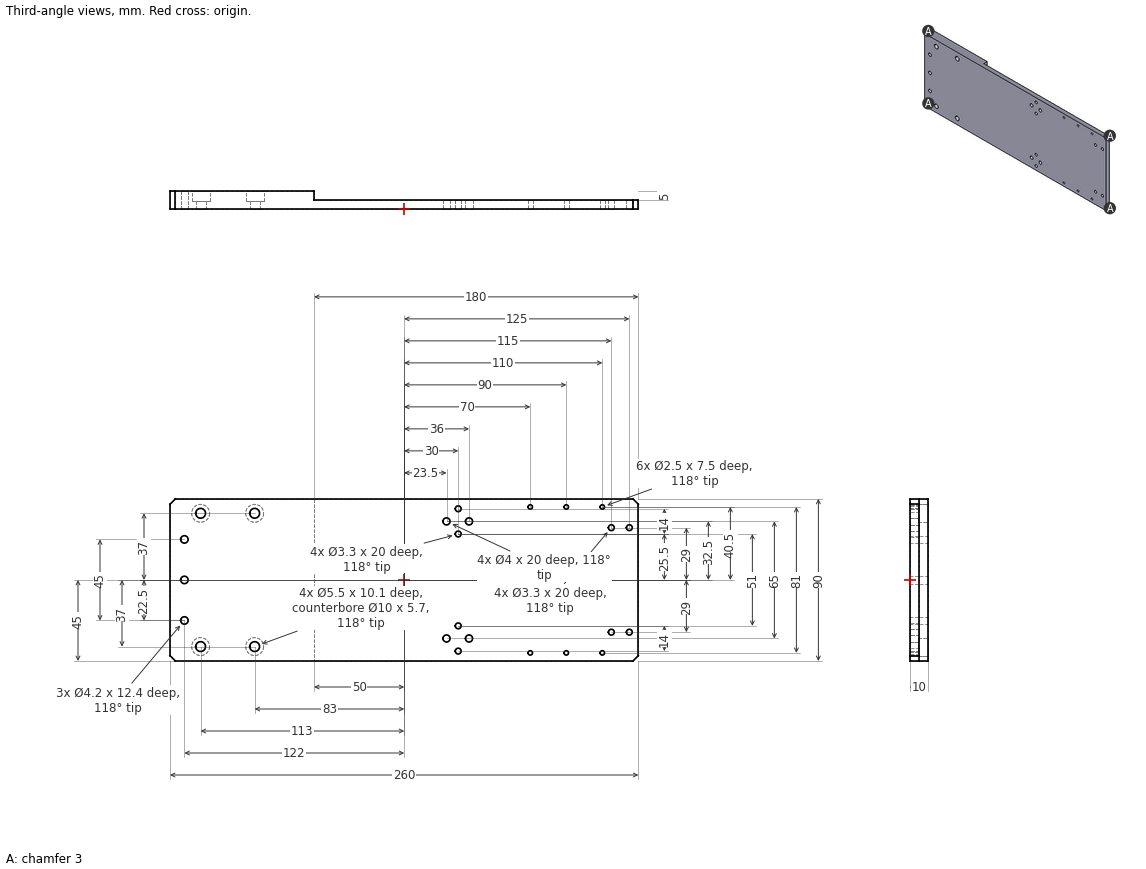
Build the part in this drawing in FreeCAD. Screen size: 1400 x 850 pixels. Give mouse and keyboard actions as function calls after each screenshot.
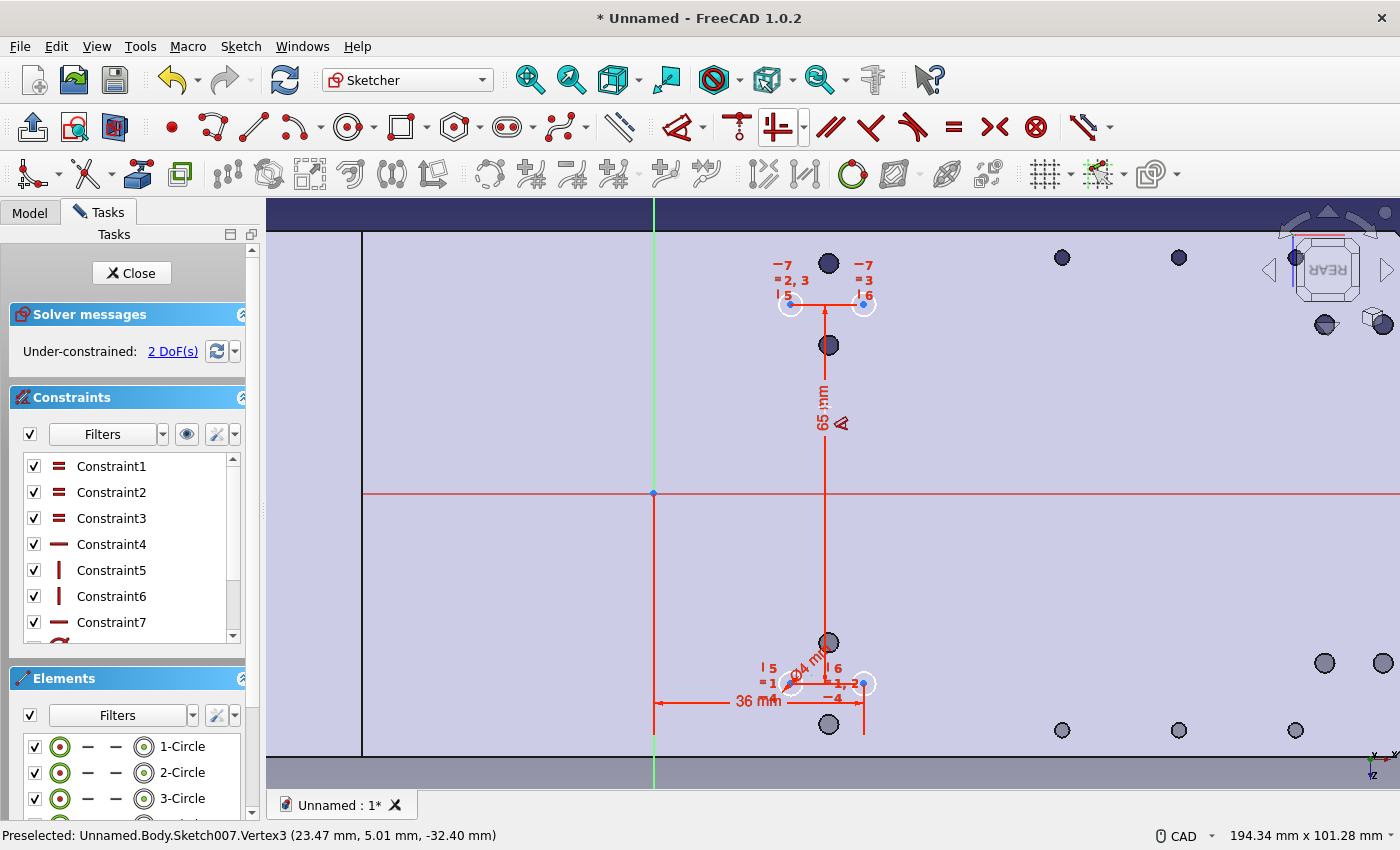
click(791, 684)
click(674, 718)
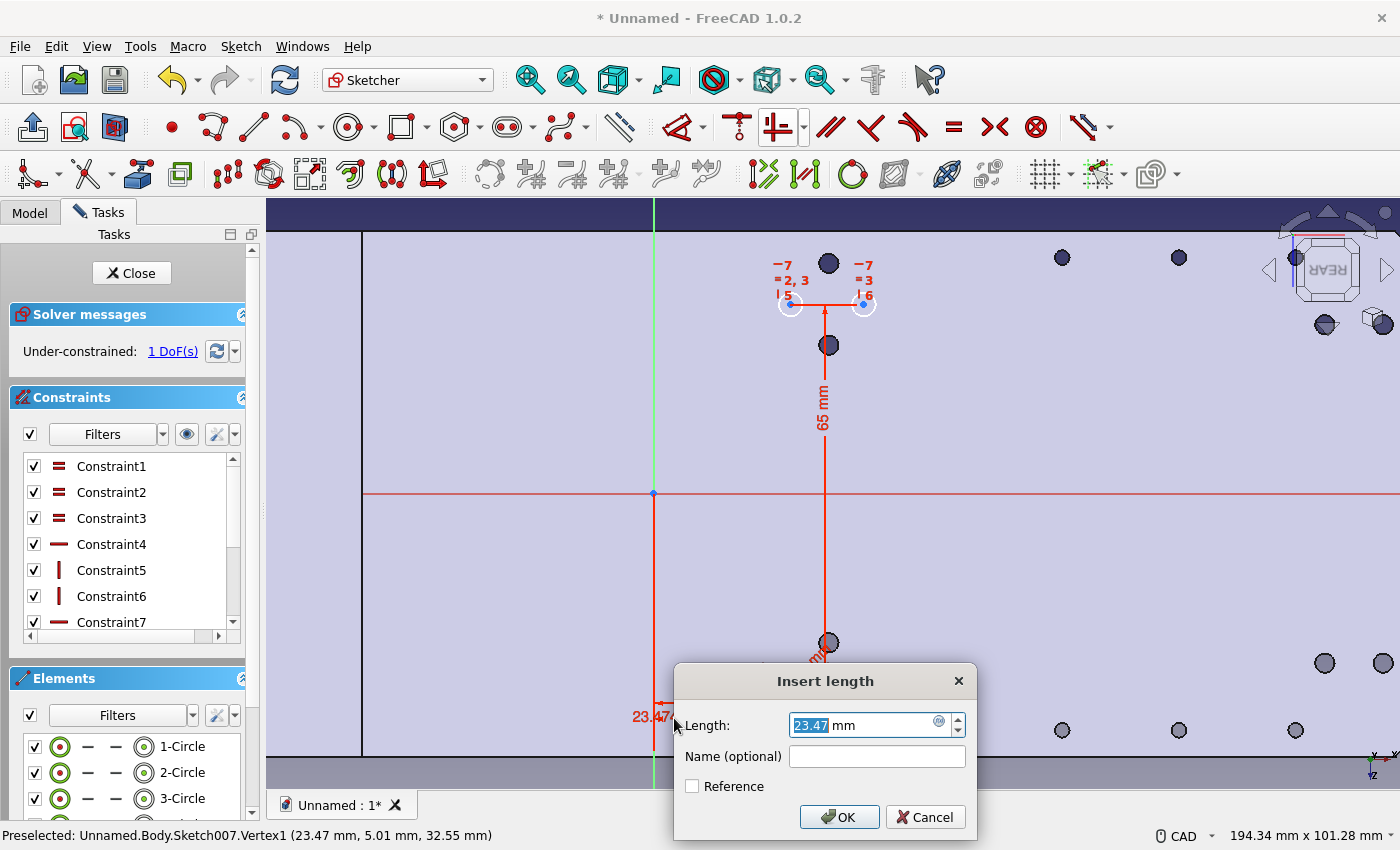
text(23.5)
key(Return)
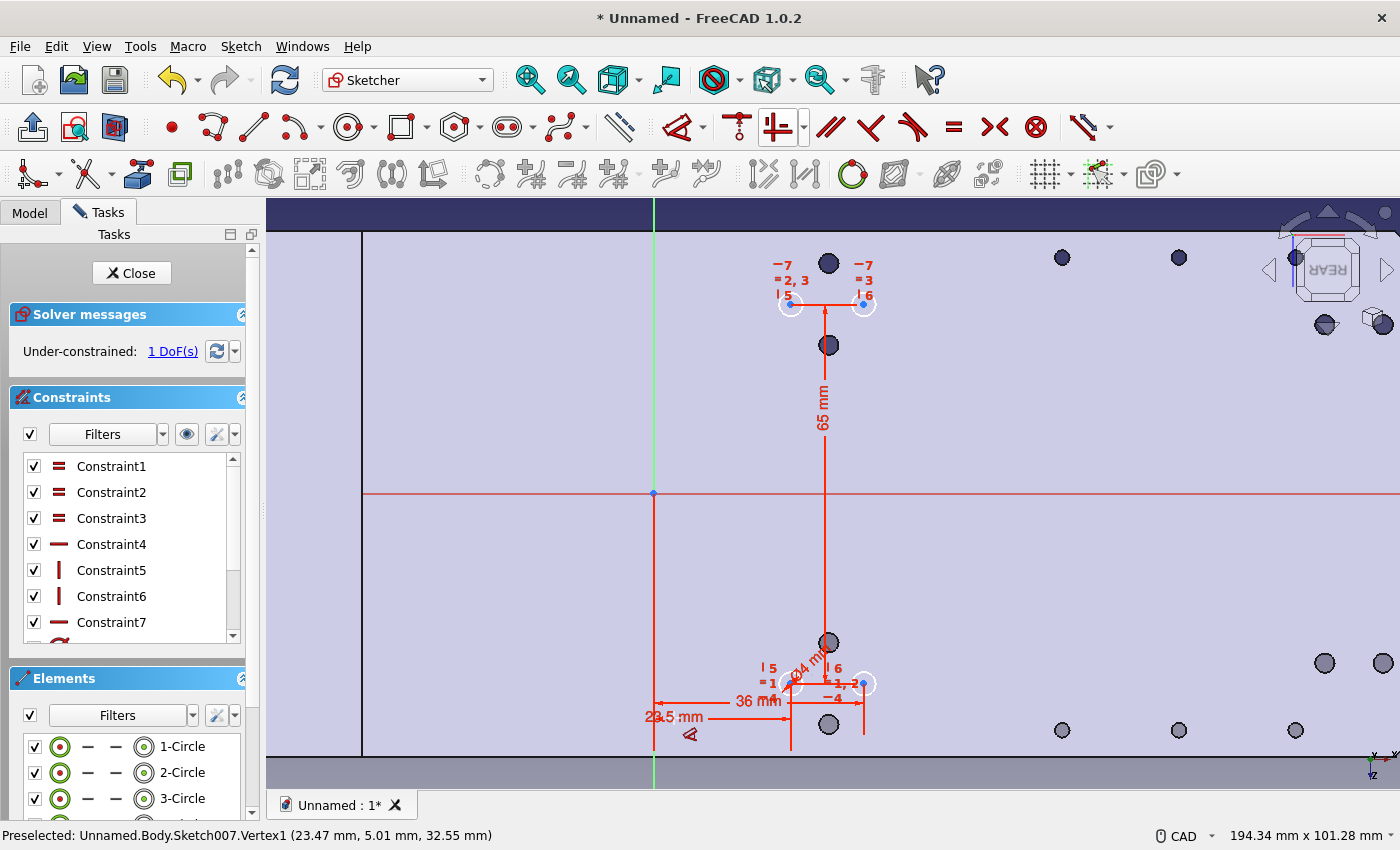
click(791, 684)
click(620, 589)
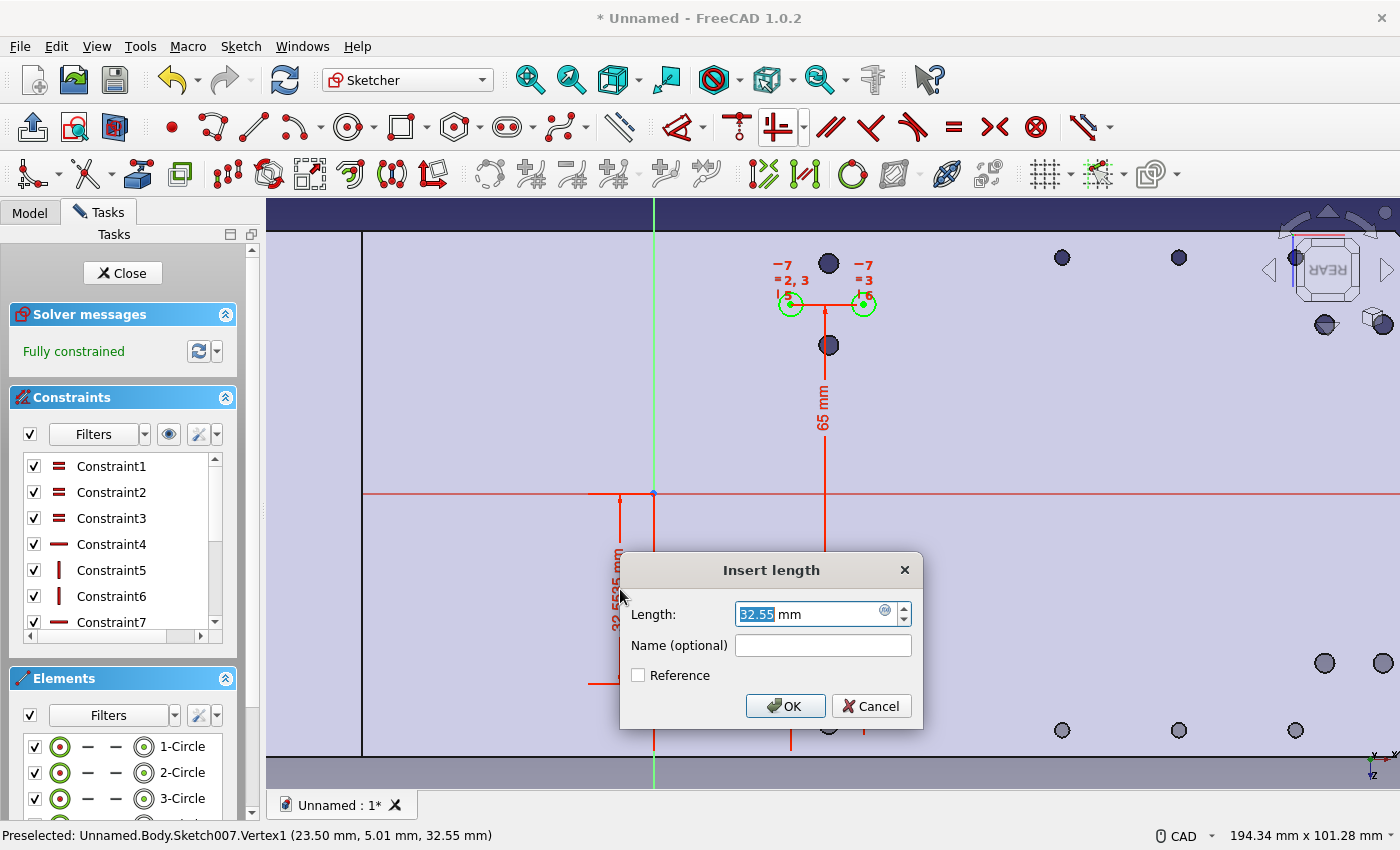
text(32.5)
key(Return)
key(Escape)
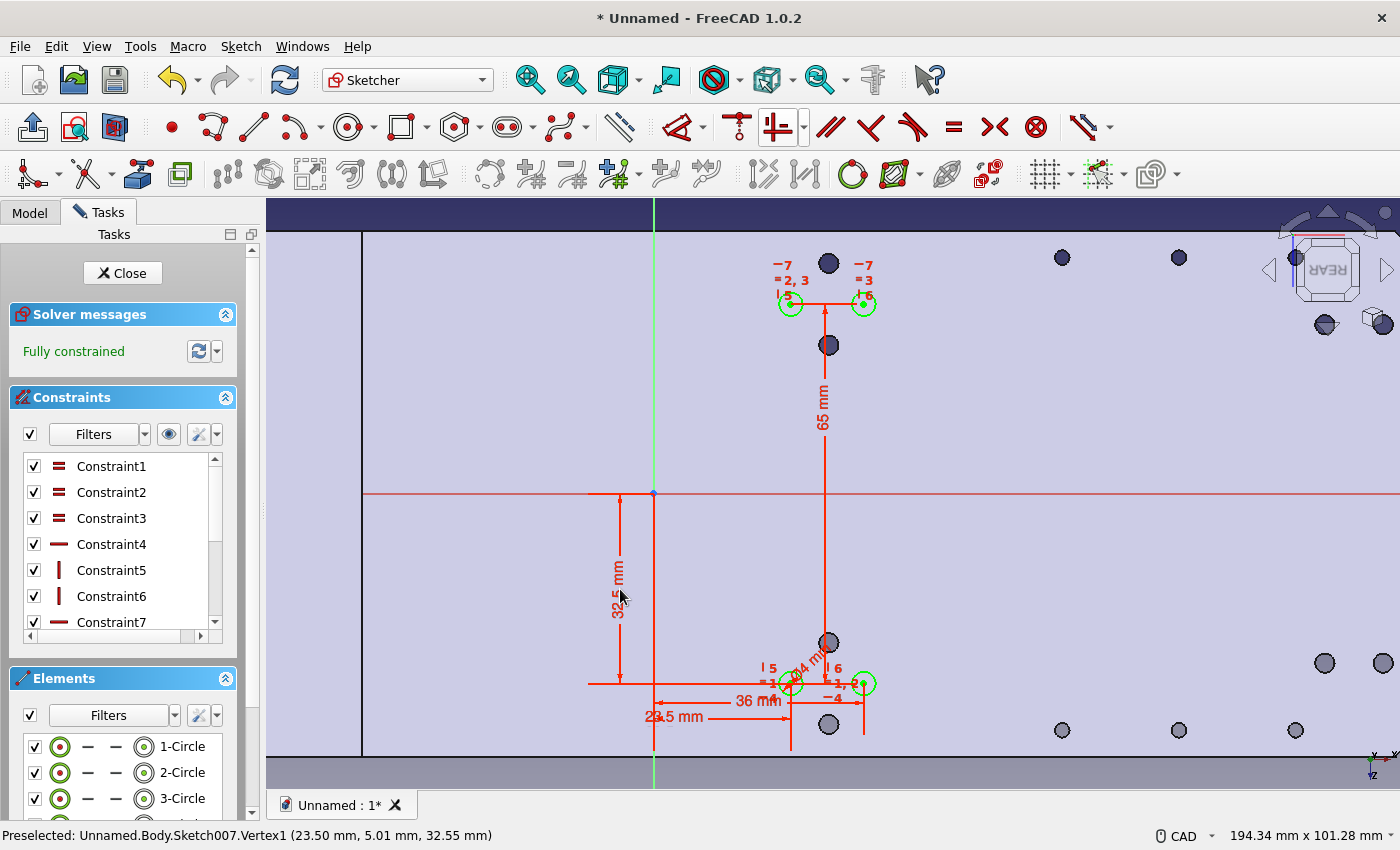
click(123, 273)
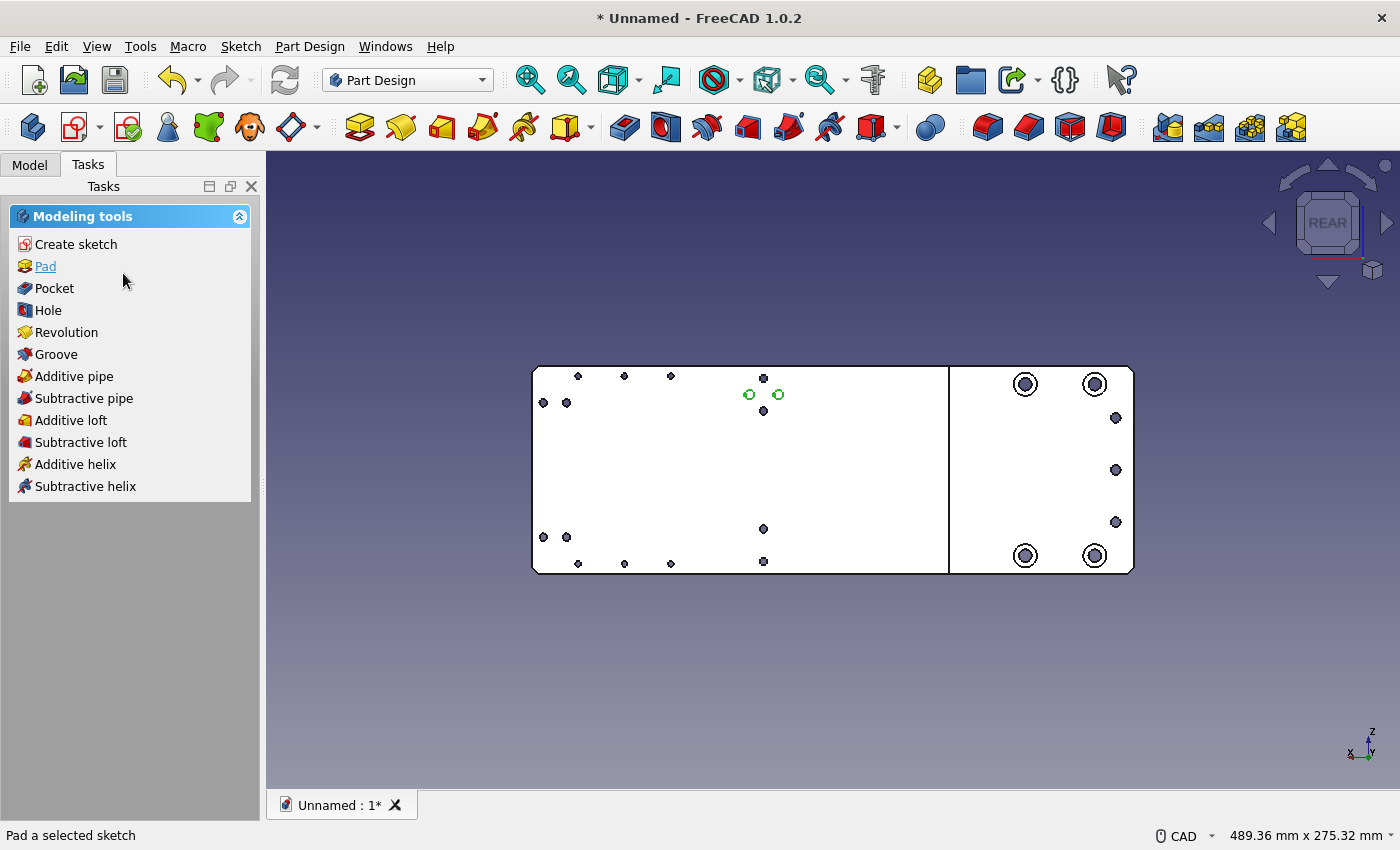
click(666, 128)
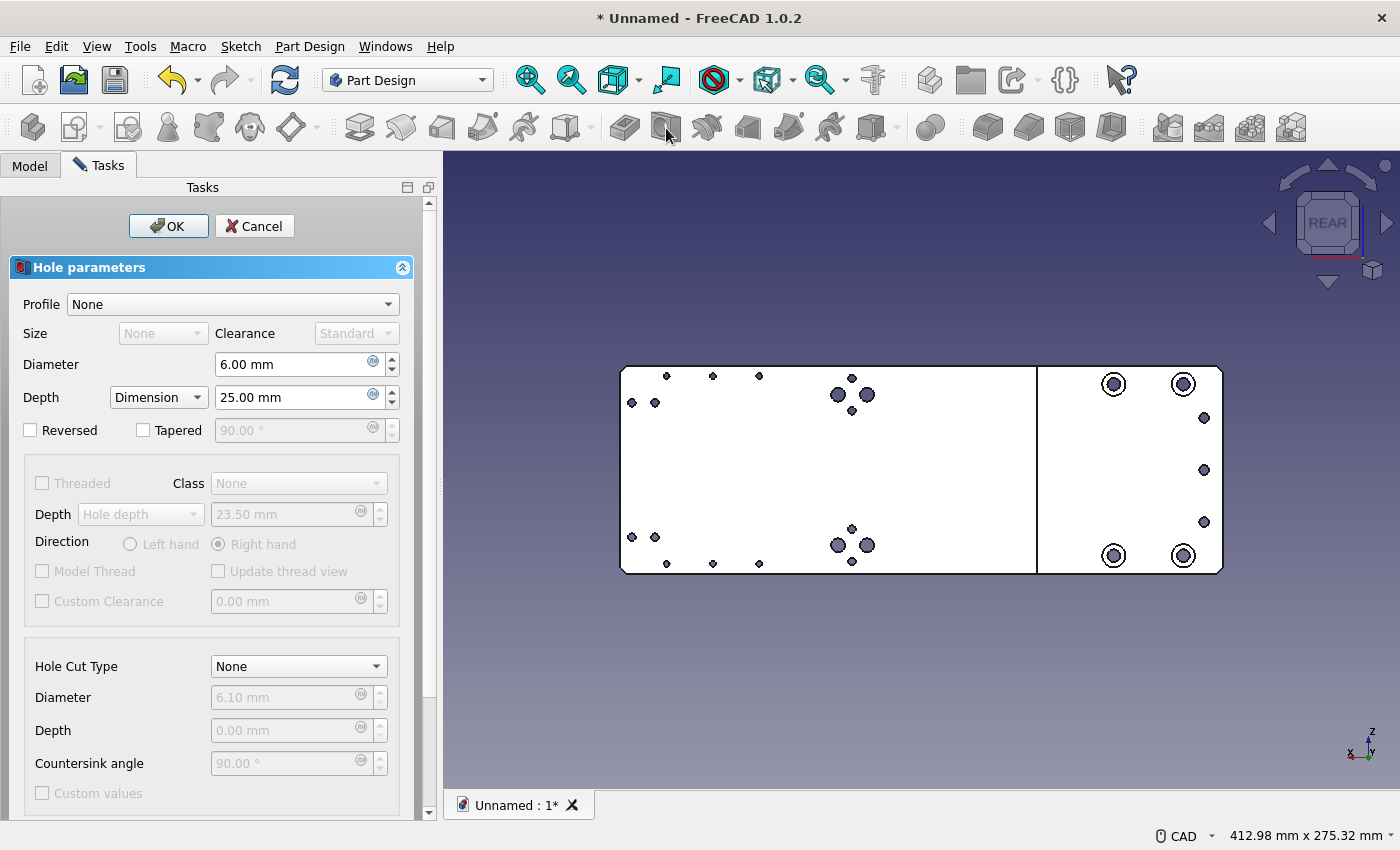
triple_click(300, 364)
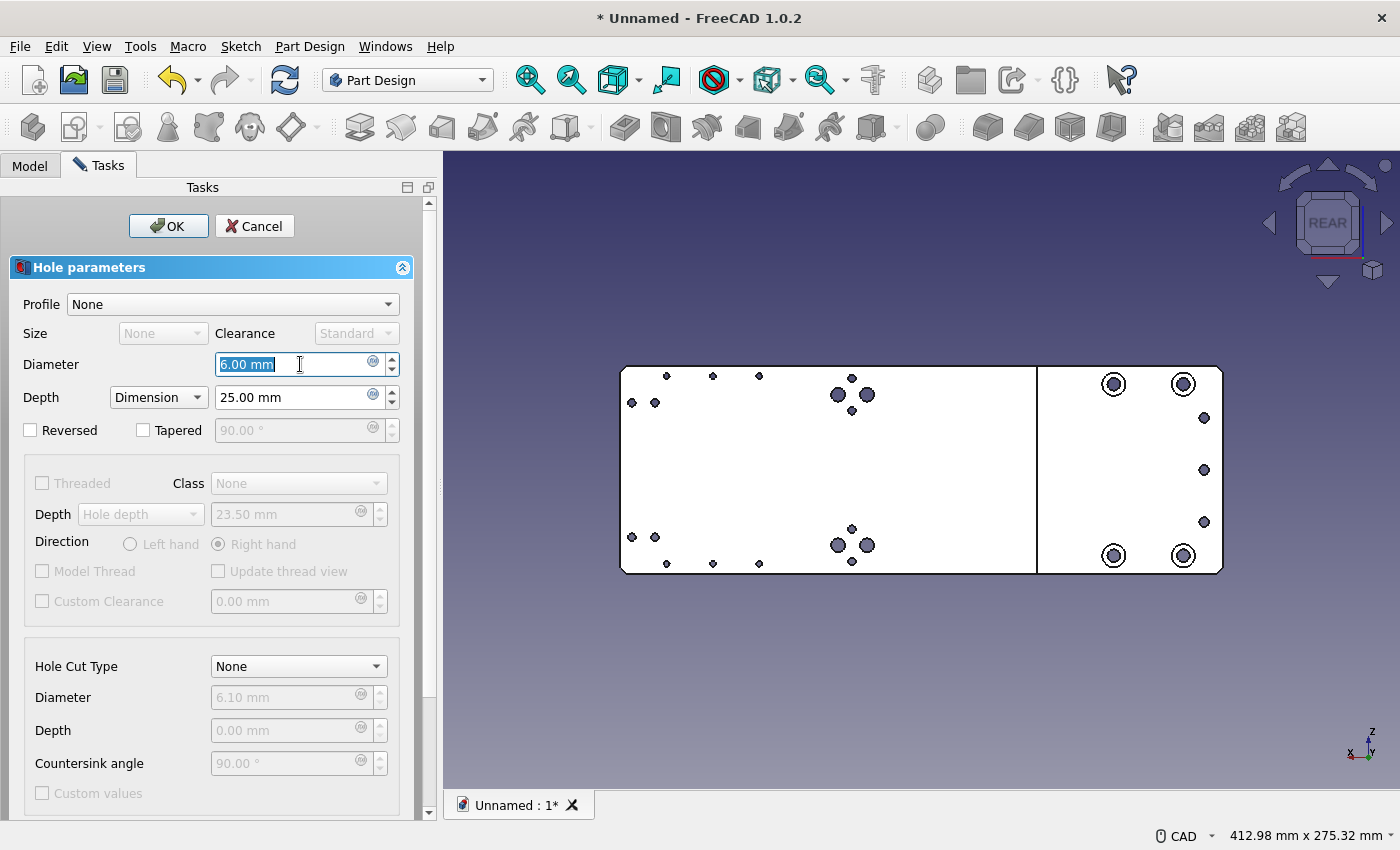
text(4)
key(Tab)